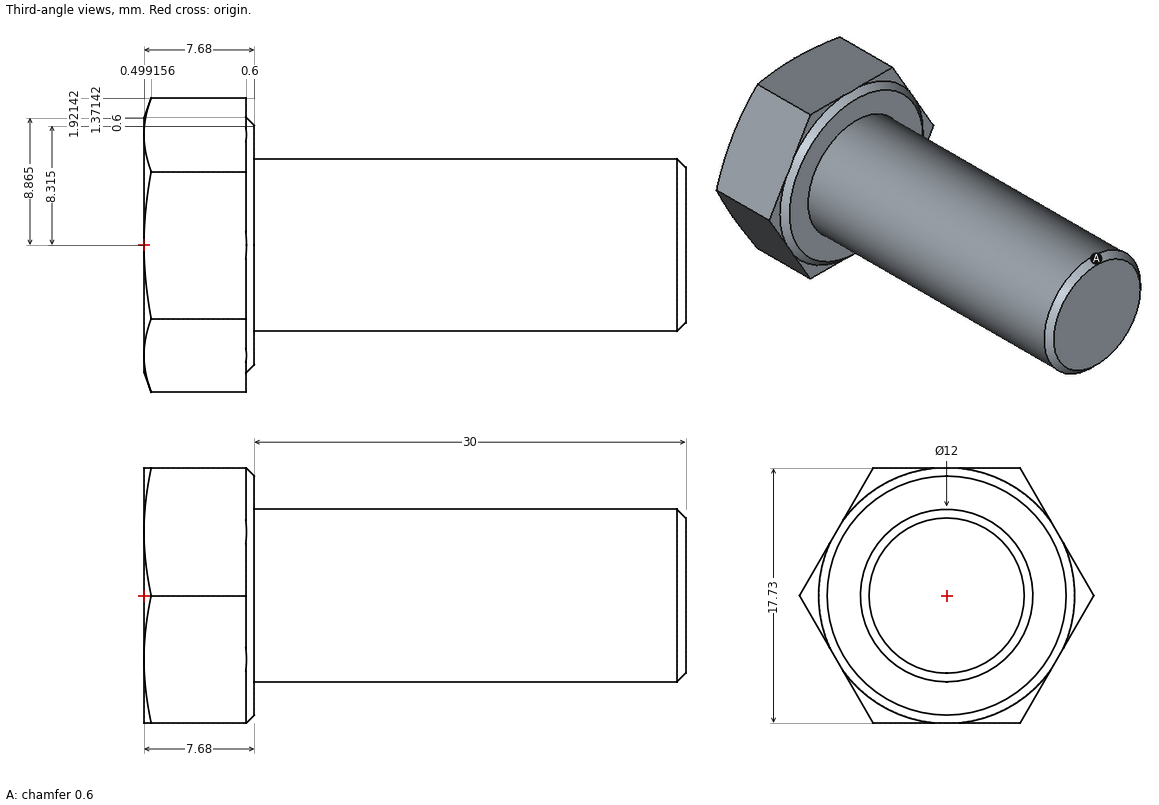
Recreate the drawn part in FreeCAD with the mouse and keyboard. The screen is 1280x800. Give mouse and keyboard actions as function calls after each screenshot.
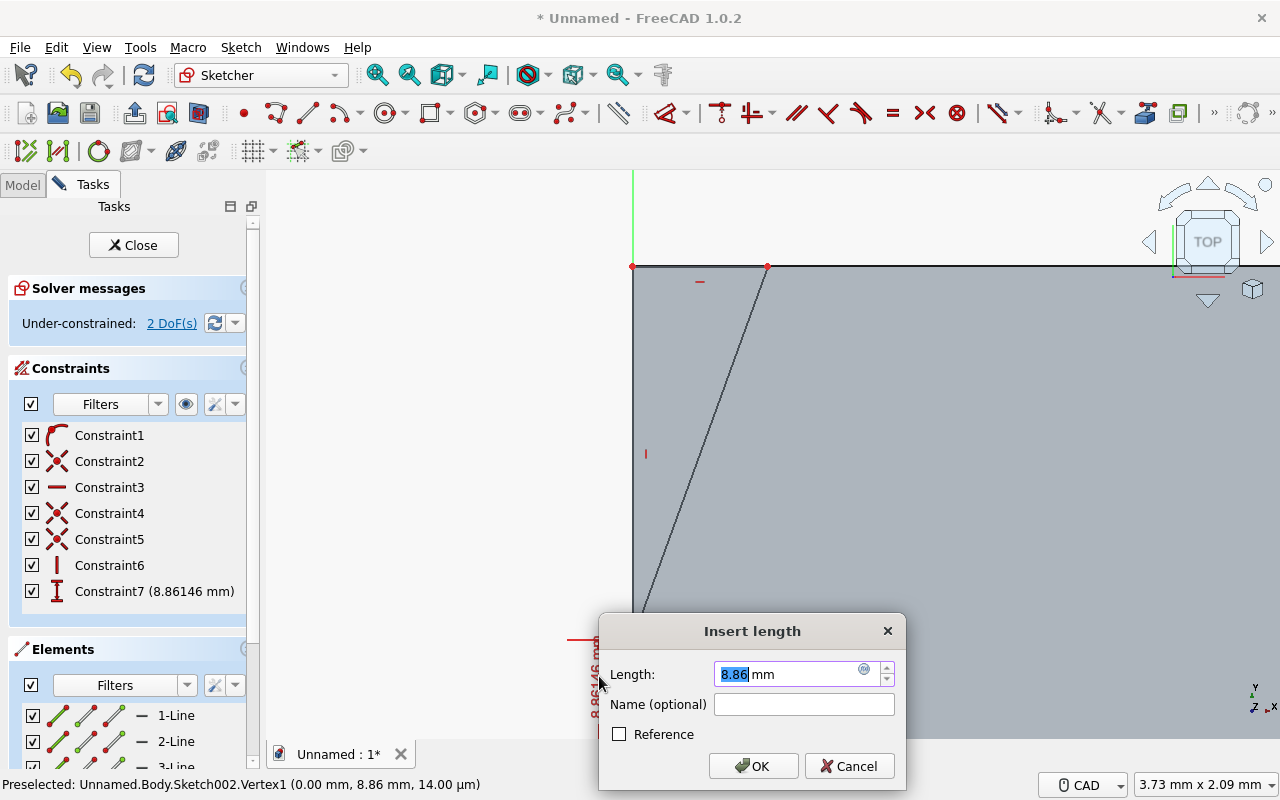
text(8.865)
key(Return)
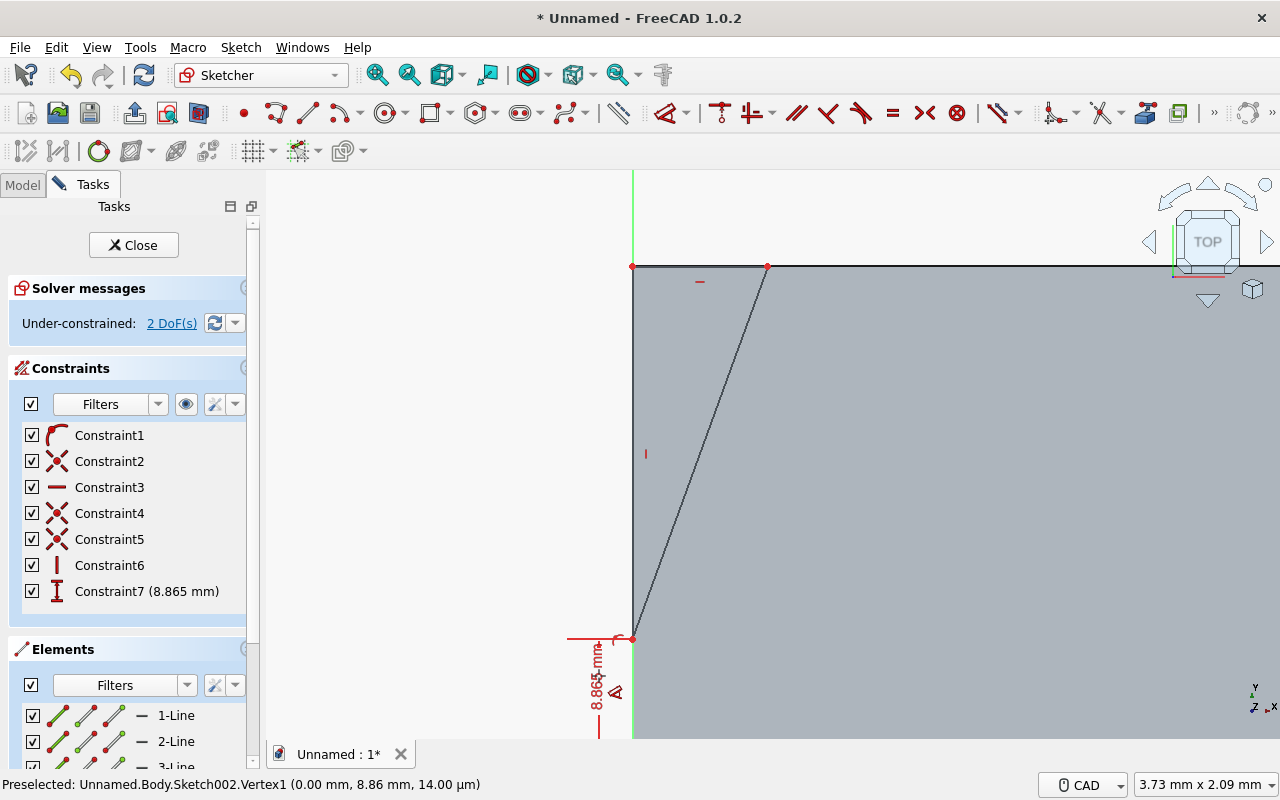
click(633, 379)
click(599, 453)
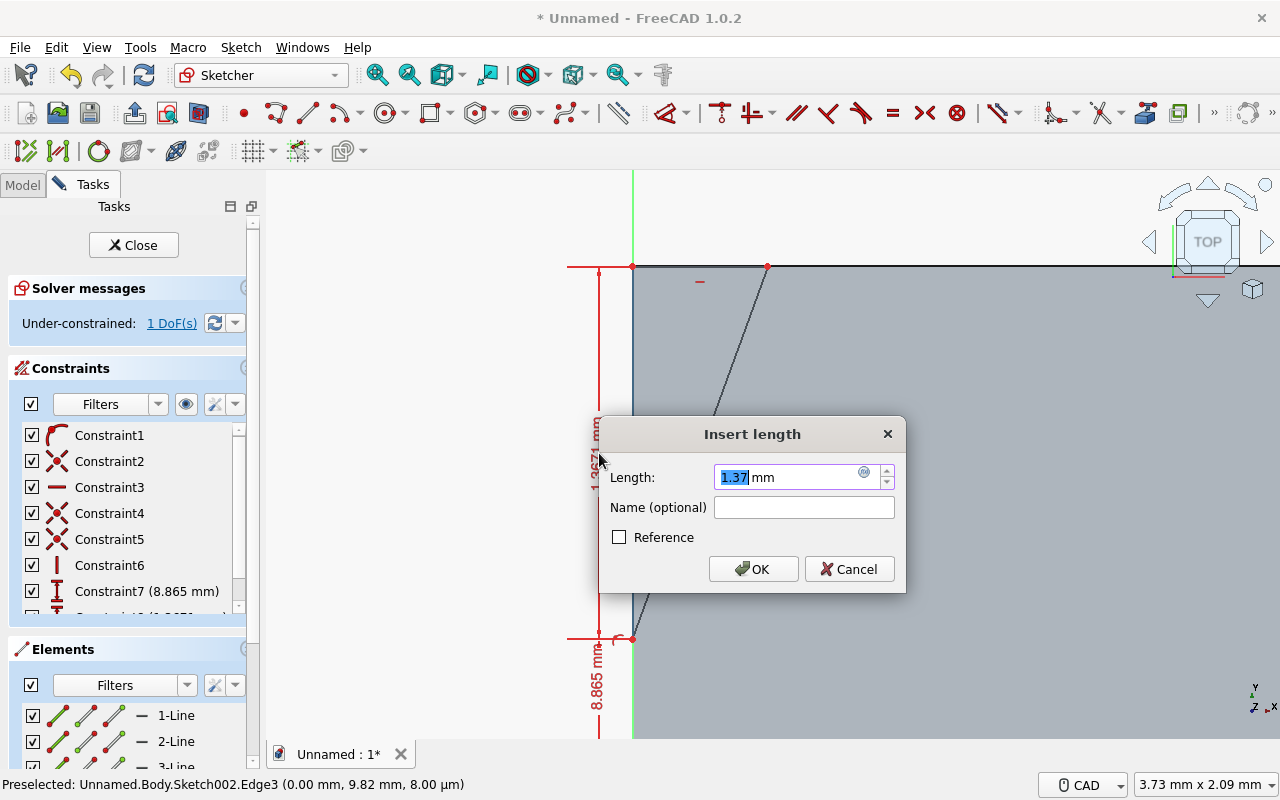
text(1.37142)
key(Return)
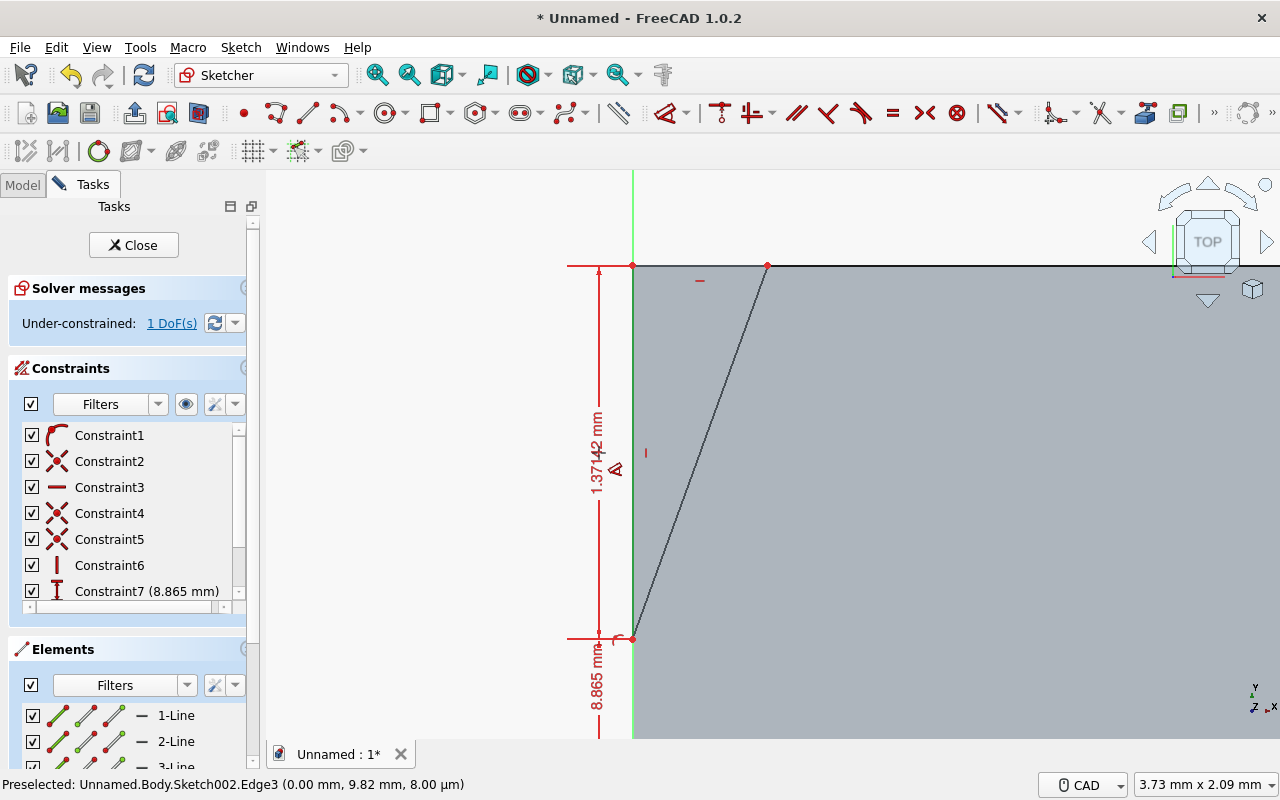
click(727, 266)
click(700, 232)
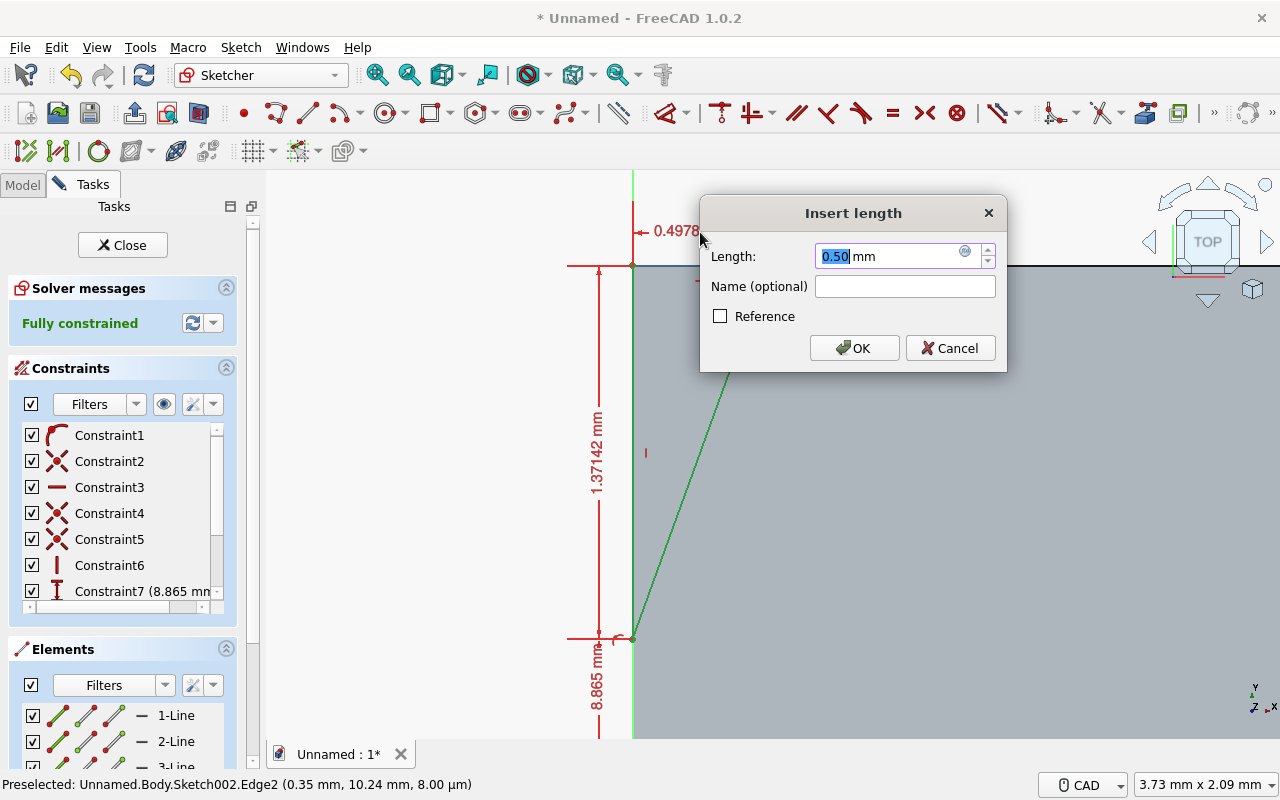
text(0.499156)
key(Return)
key(Escape)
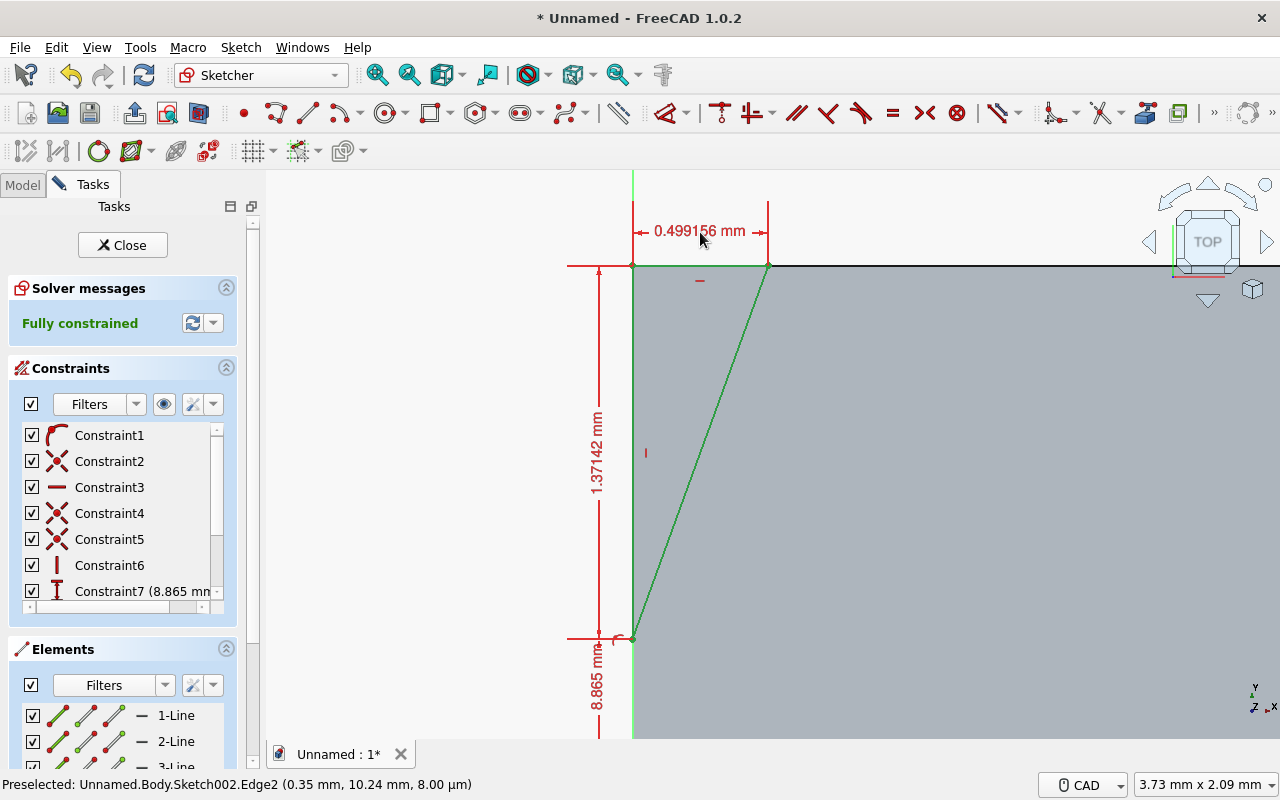
click(123, 245)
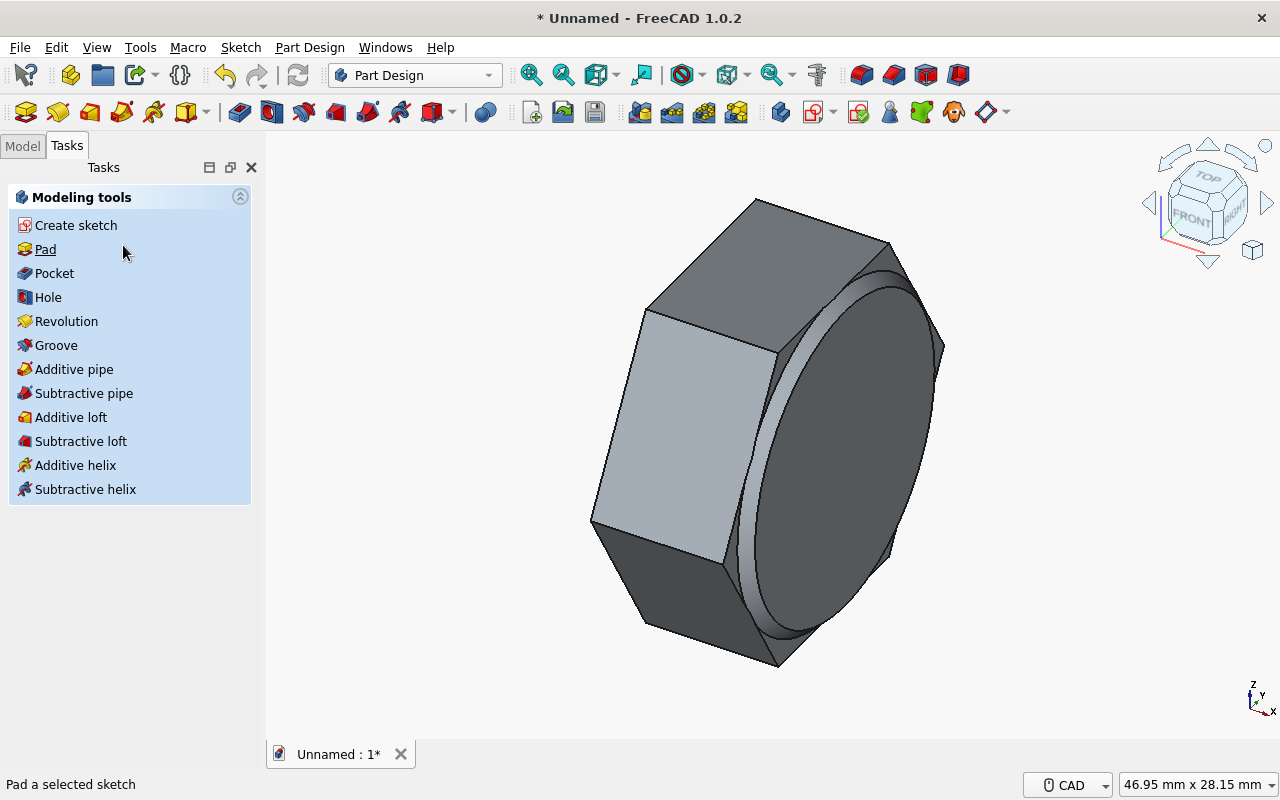
click(304, 112)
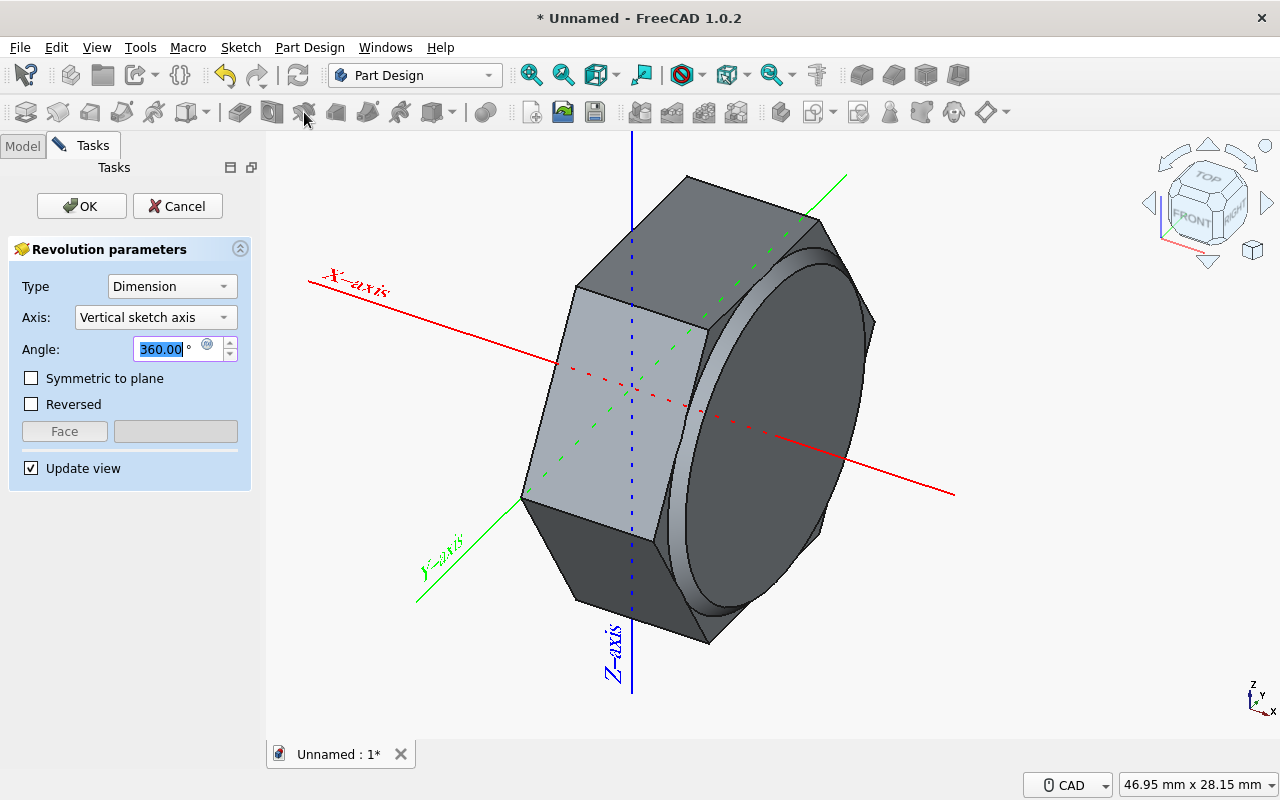
click(156, 318)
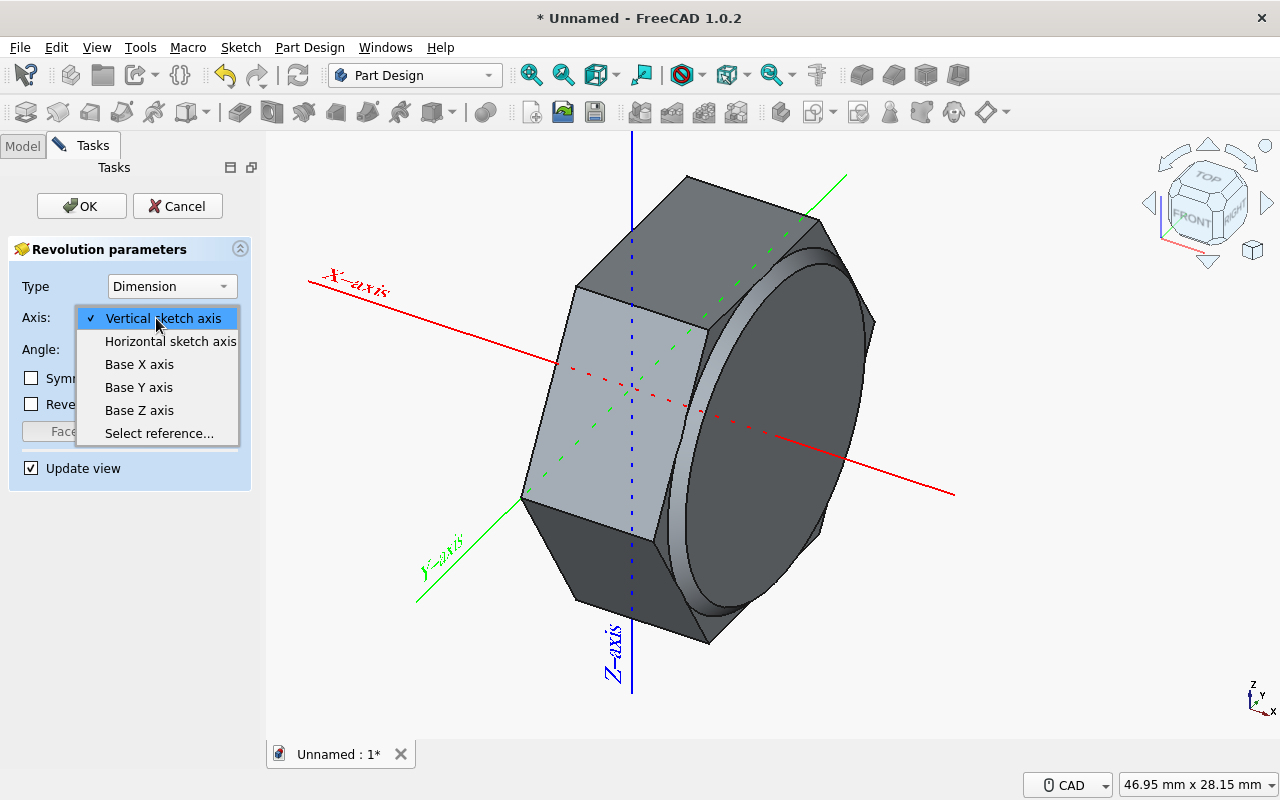
click(156, 342)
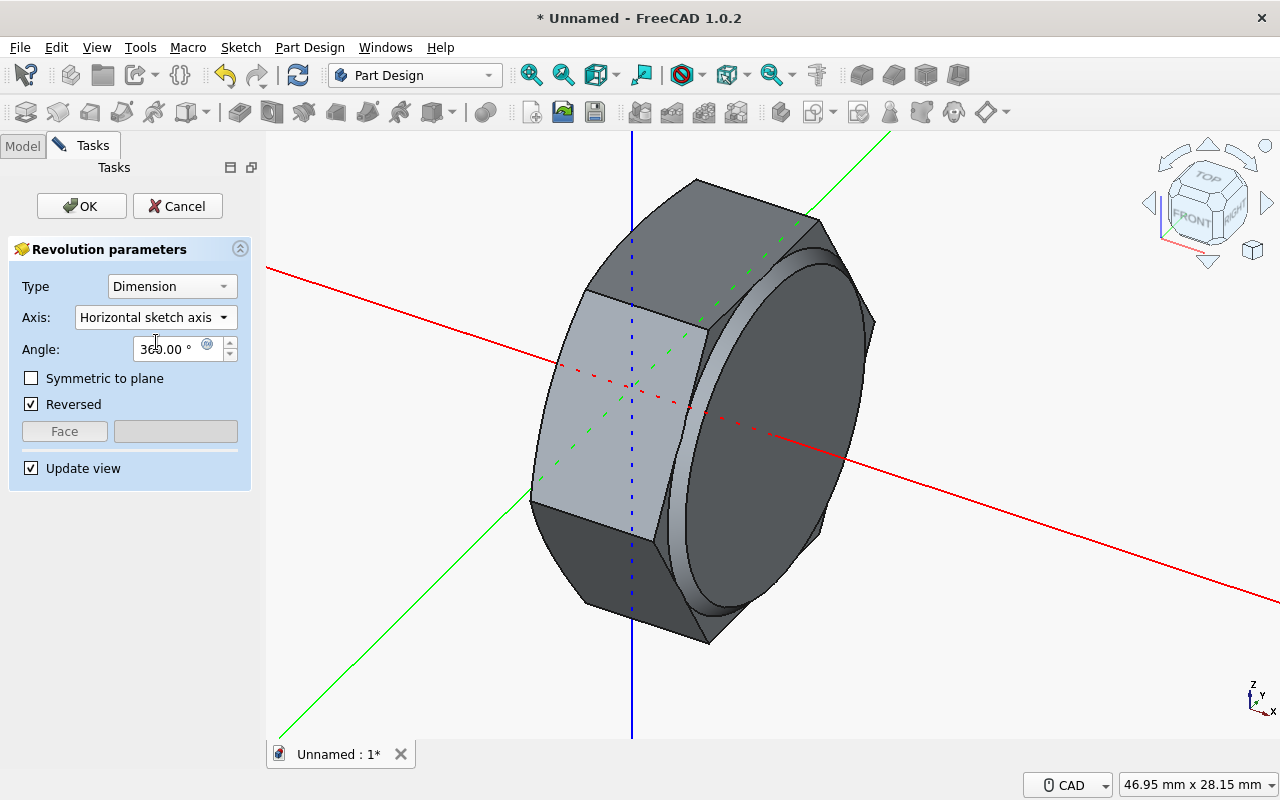
click(82, 206)